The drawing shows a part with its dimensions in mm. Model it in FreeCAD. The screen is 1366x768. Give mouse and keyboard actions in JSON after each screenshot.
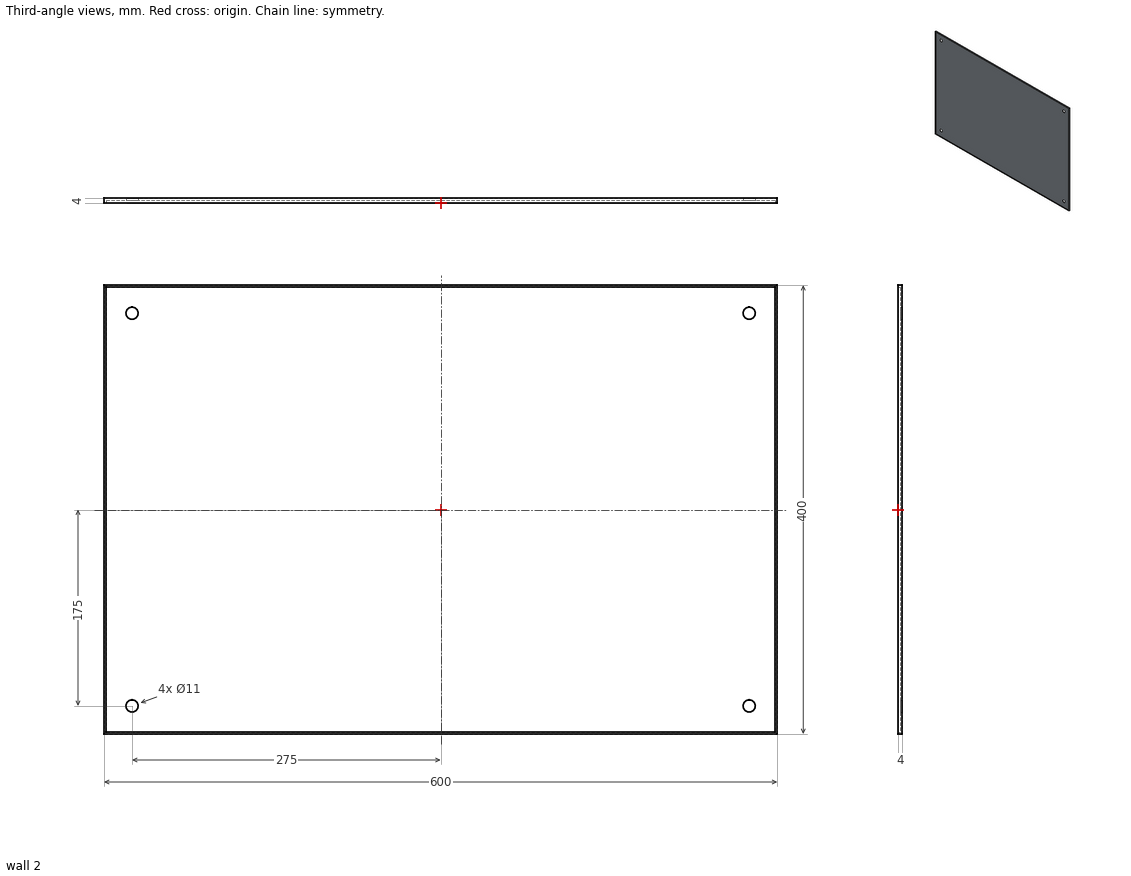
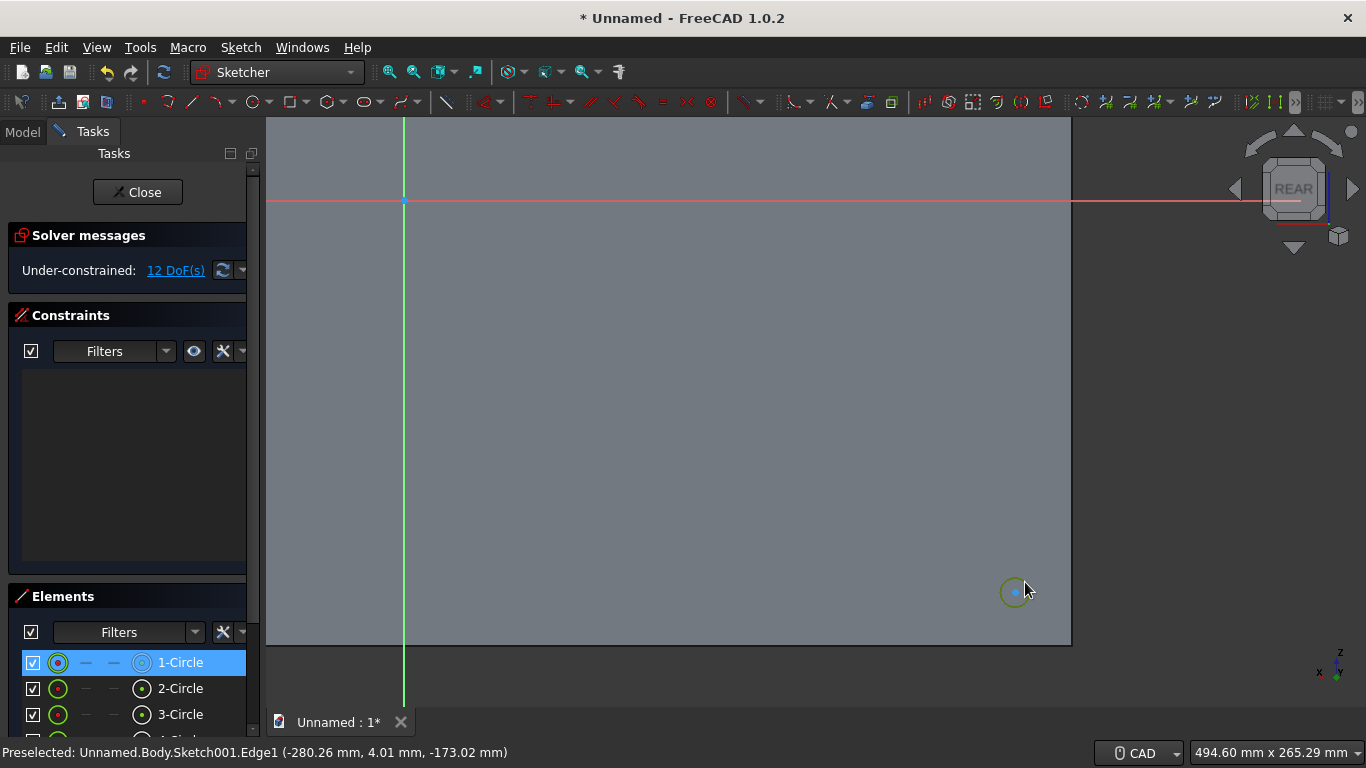
{"action": "scroll", "coordinate": [1027, 584], "scroll_direction": "down", "scroll_amount": 4}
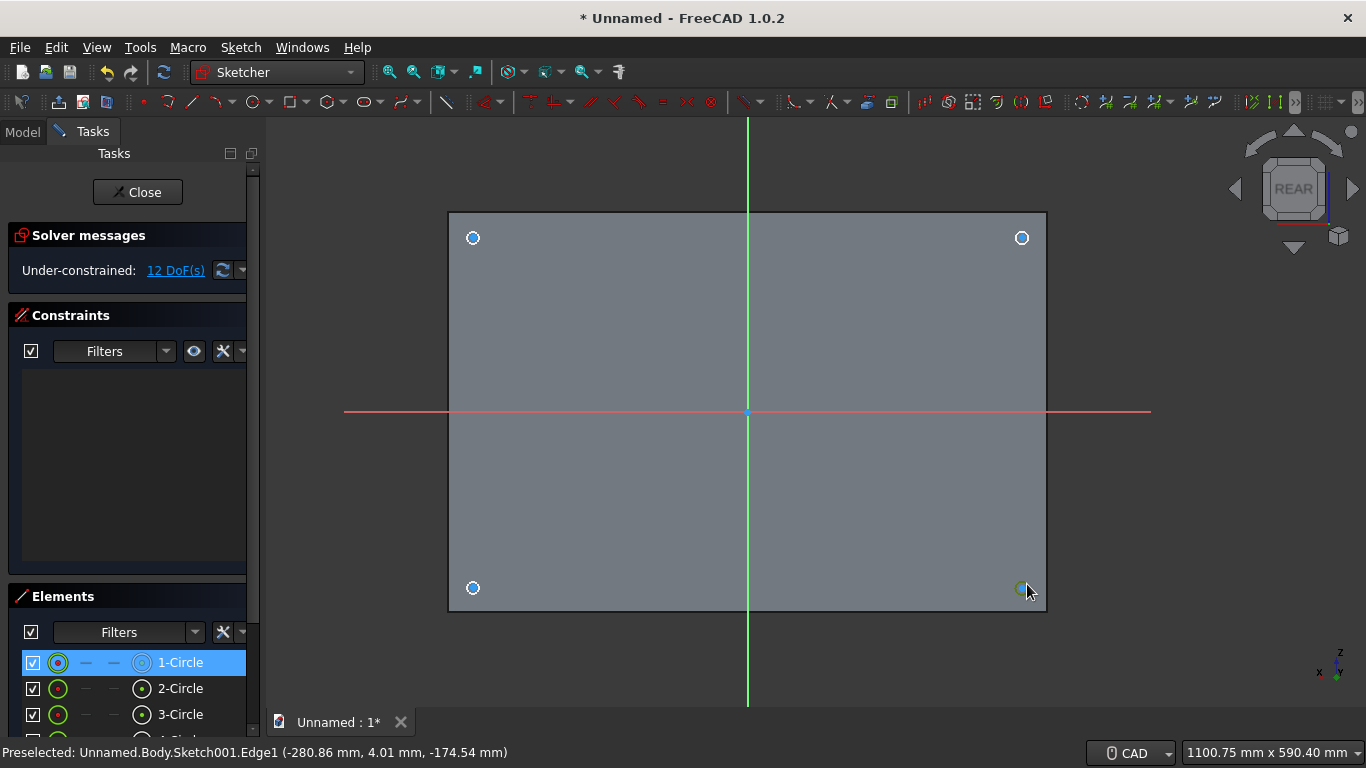
{"action": "scroll", "coordinate": [477, 584], "scroll_direction": "up", "scroll_amount": 5}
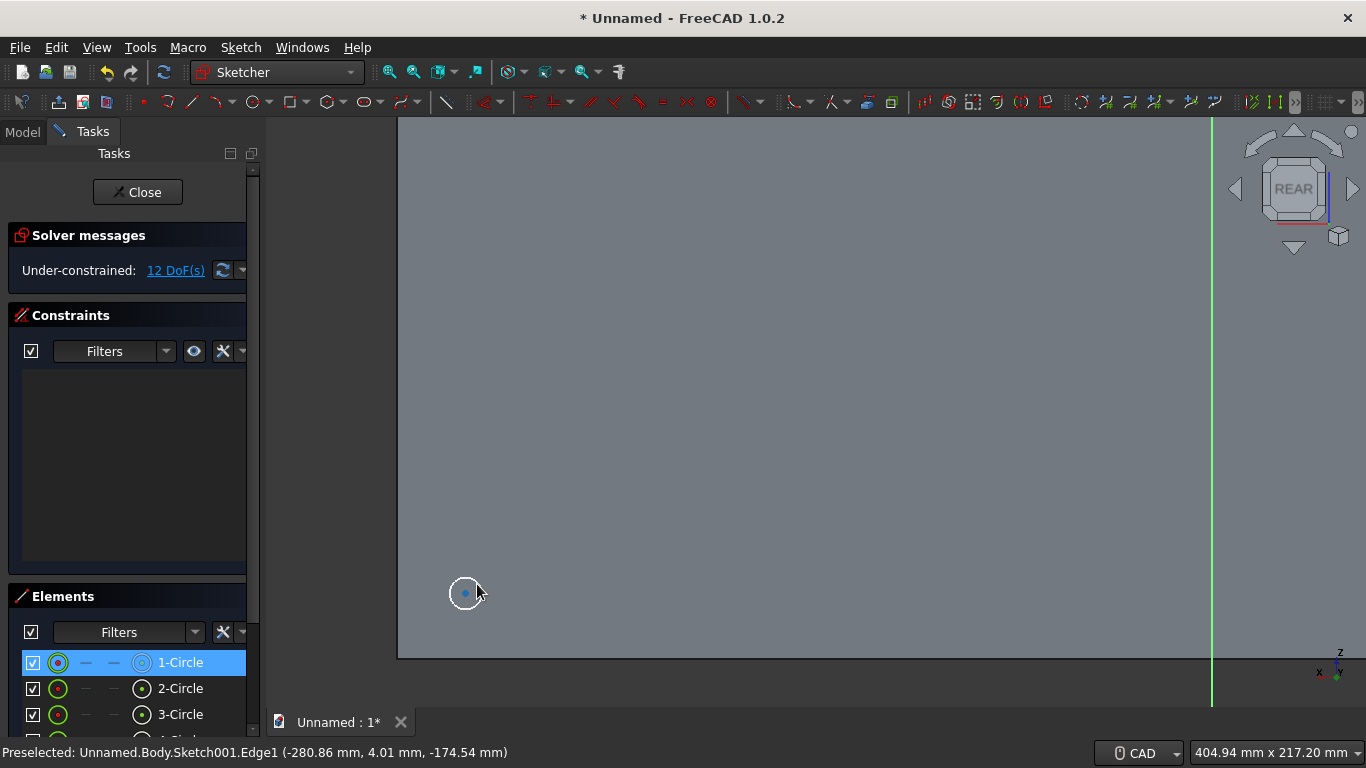
{"action": "left_click", "coordinate": [477, 582]}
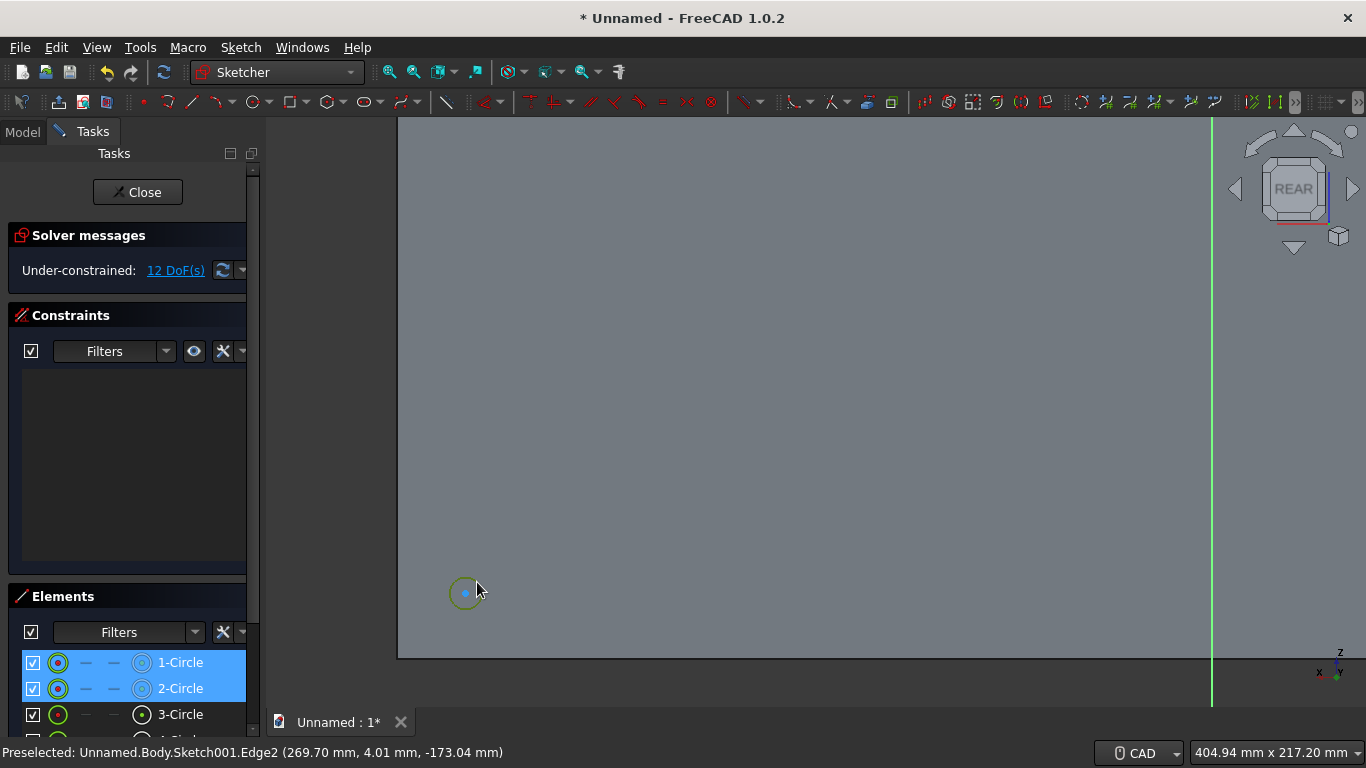
{"action": "scroll", "coordinate": [477, 584], "scroll_direction": "down", "scroll_amount": 5}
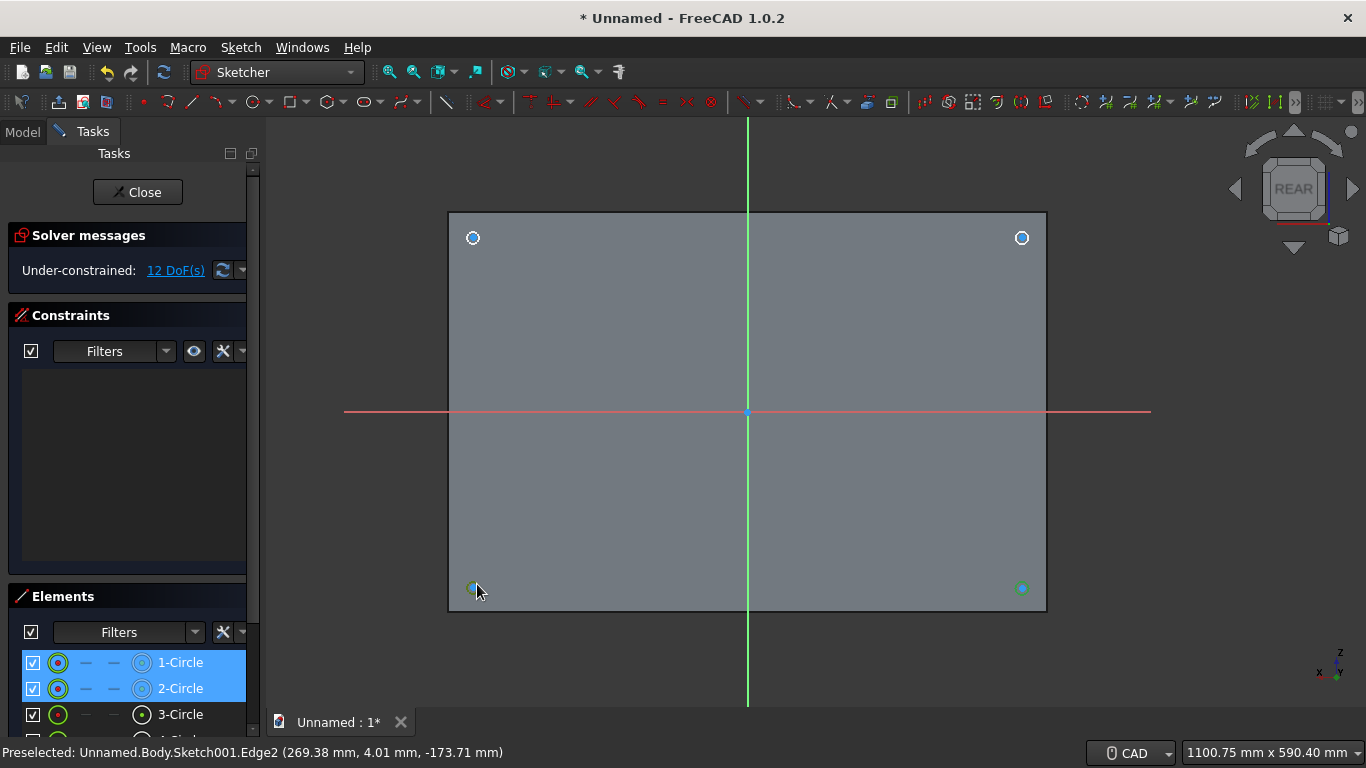
{"action": "scroll", "coordinate": [477, 234], "scroll_direction": "up", "scroll_amount": 5}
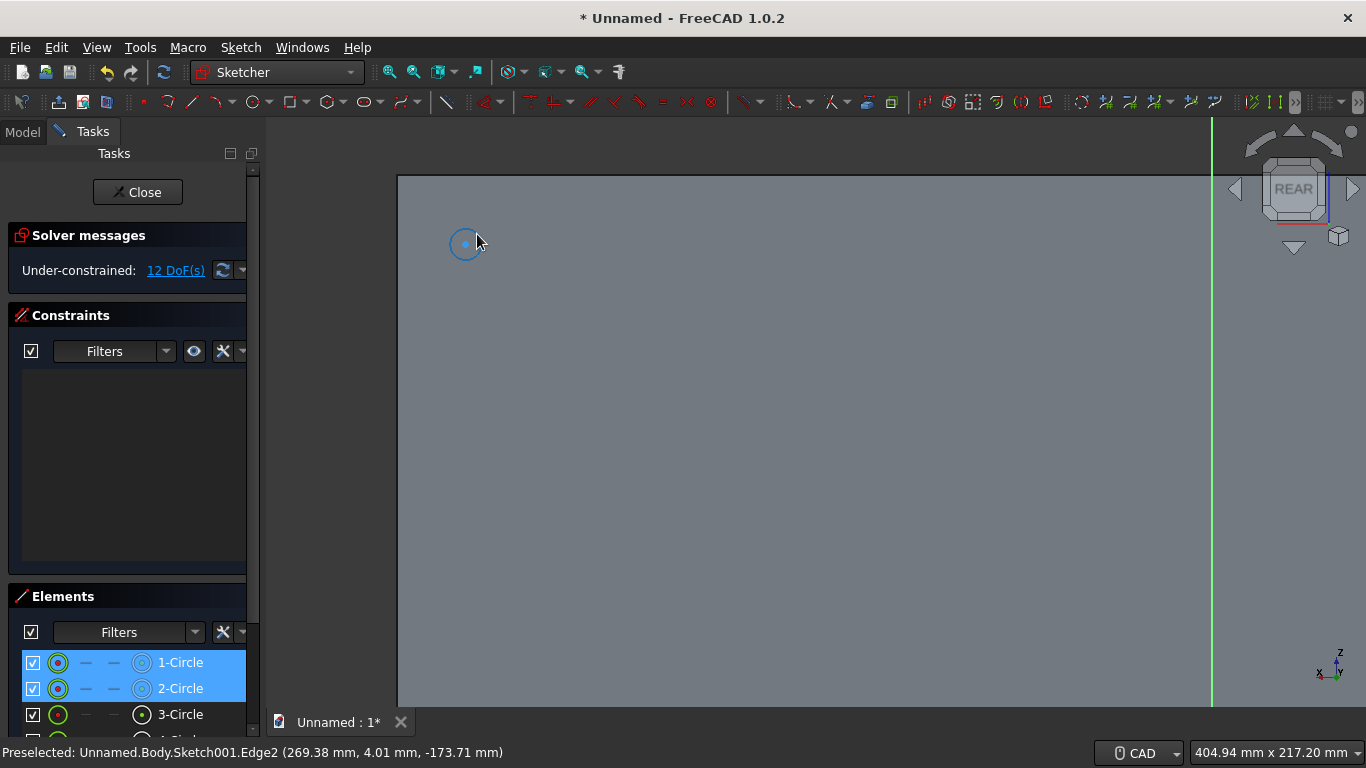
{"action": "left_click", "coordinate": [477, 233]}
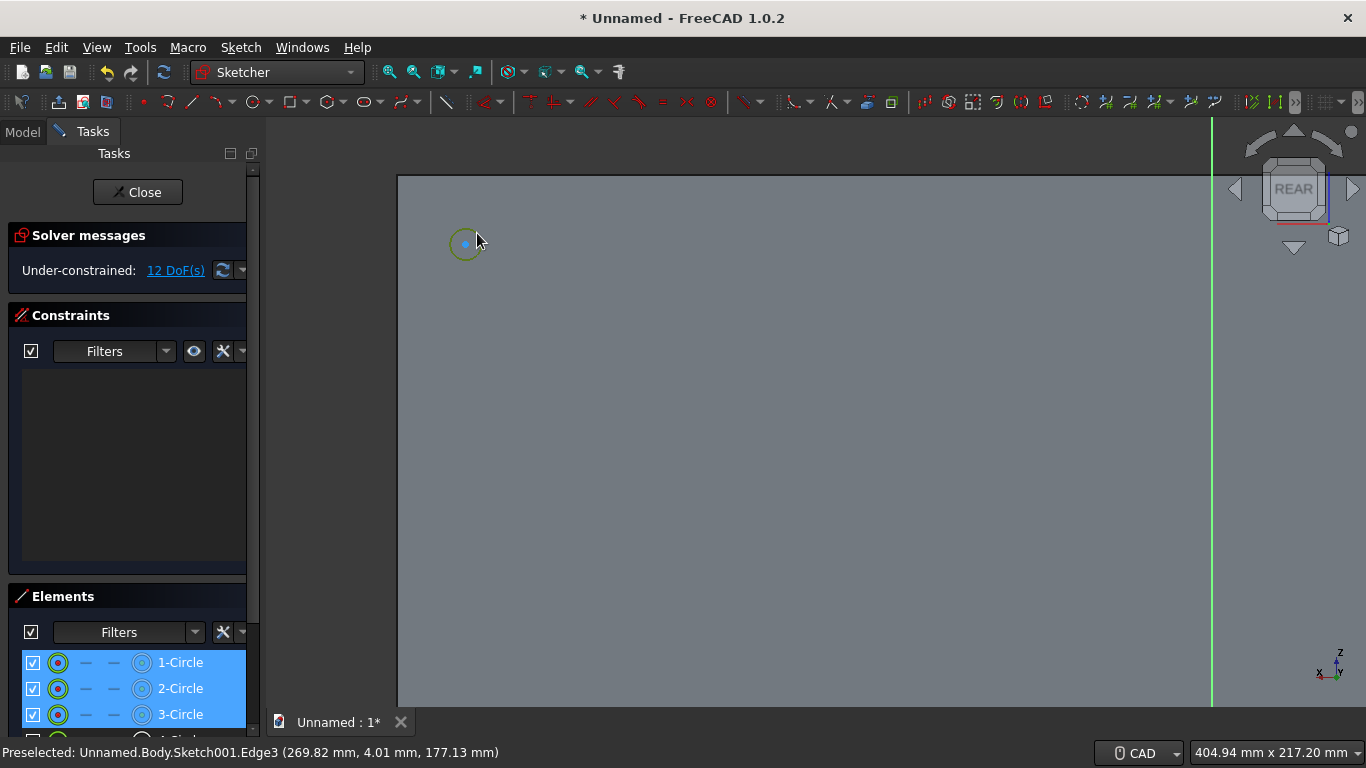
{"action": "scroll", "coordinate": [477, 234], "scroll_direction": "down", "scroll_amount": 5}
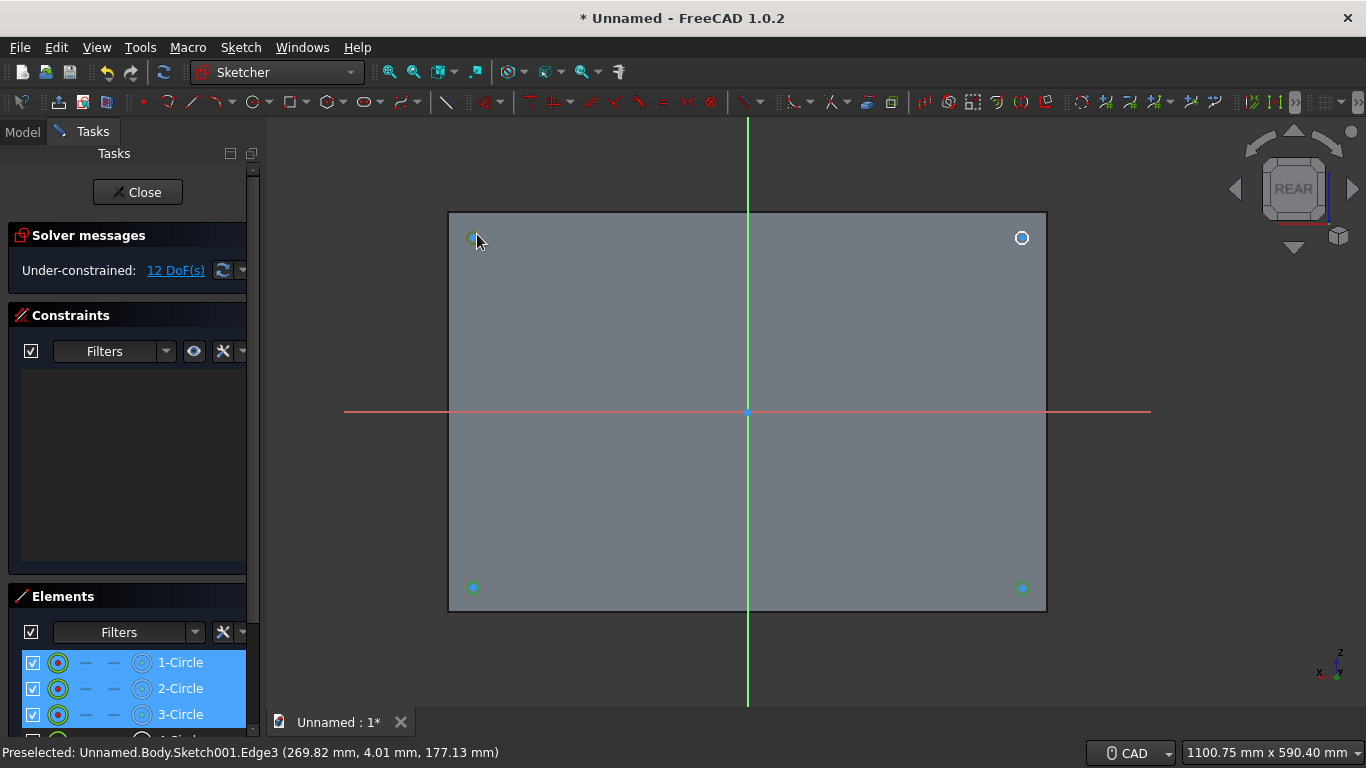
{"action": "scroll", "coordinate": [1026, 234], "scroll_direction": "up", "scroll_amount": 5}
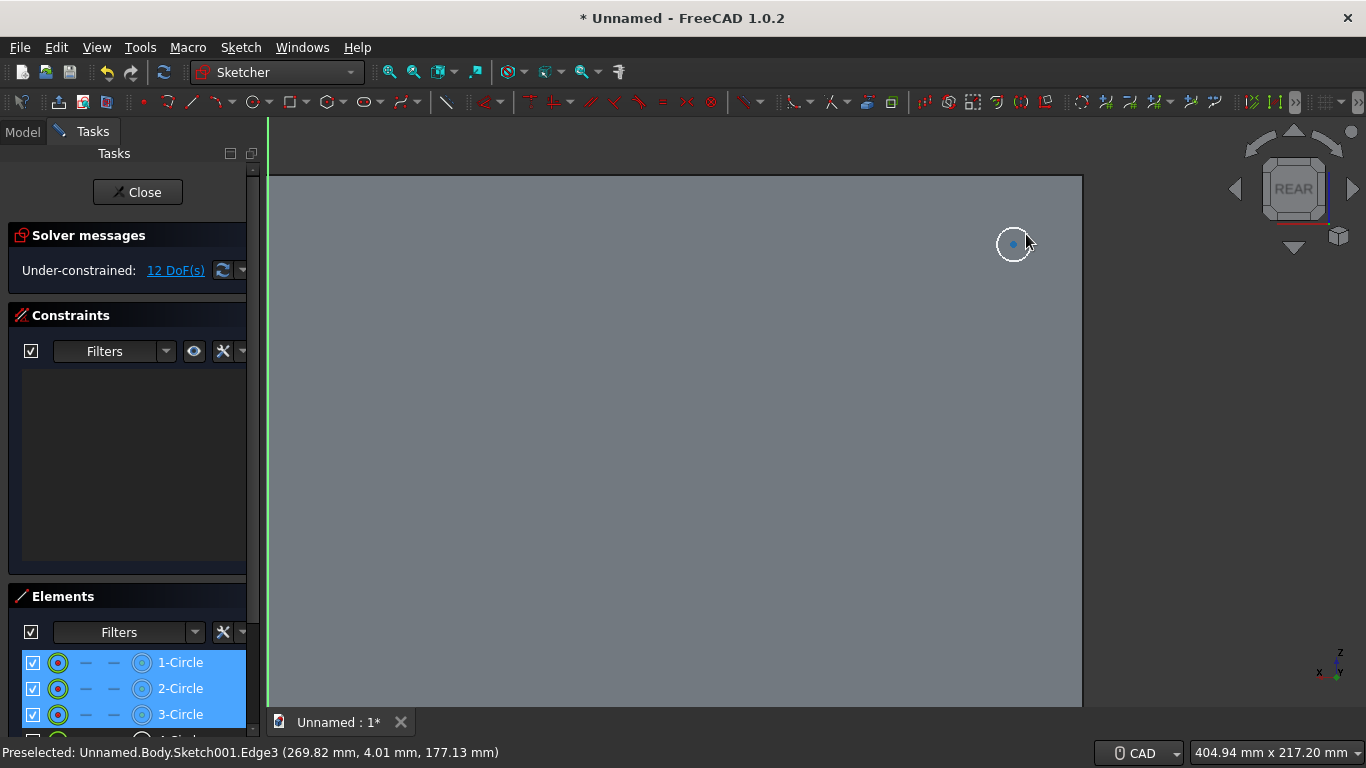
{"action": "left_click", "coordinate": [1026, 233]}